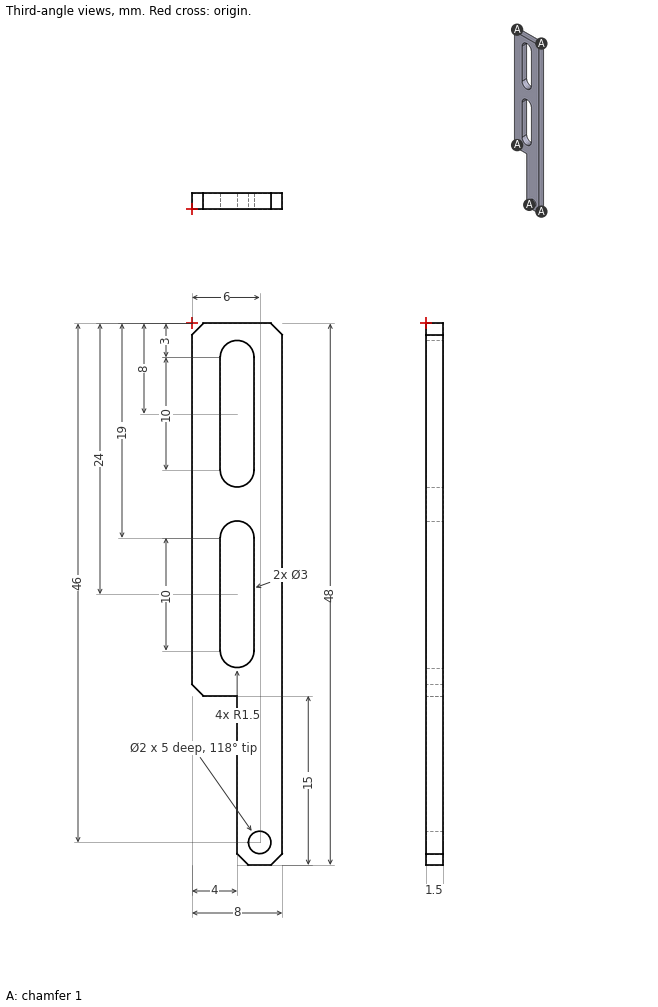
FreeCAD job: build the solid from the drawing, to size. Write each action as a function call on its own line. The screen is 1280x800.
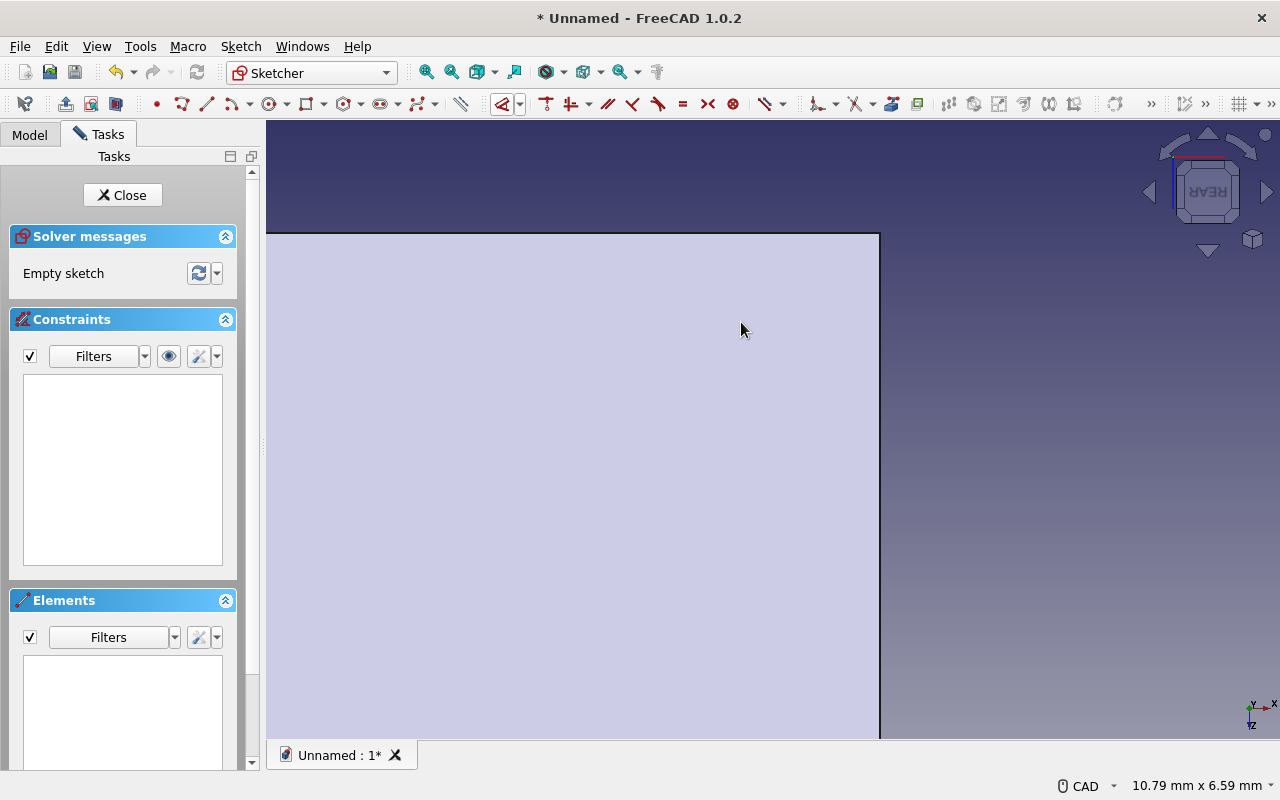
scroll(682, 414, up, 4)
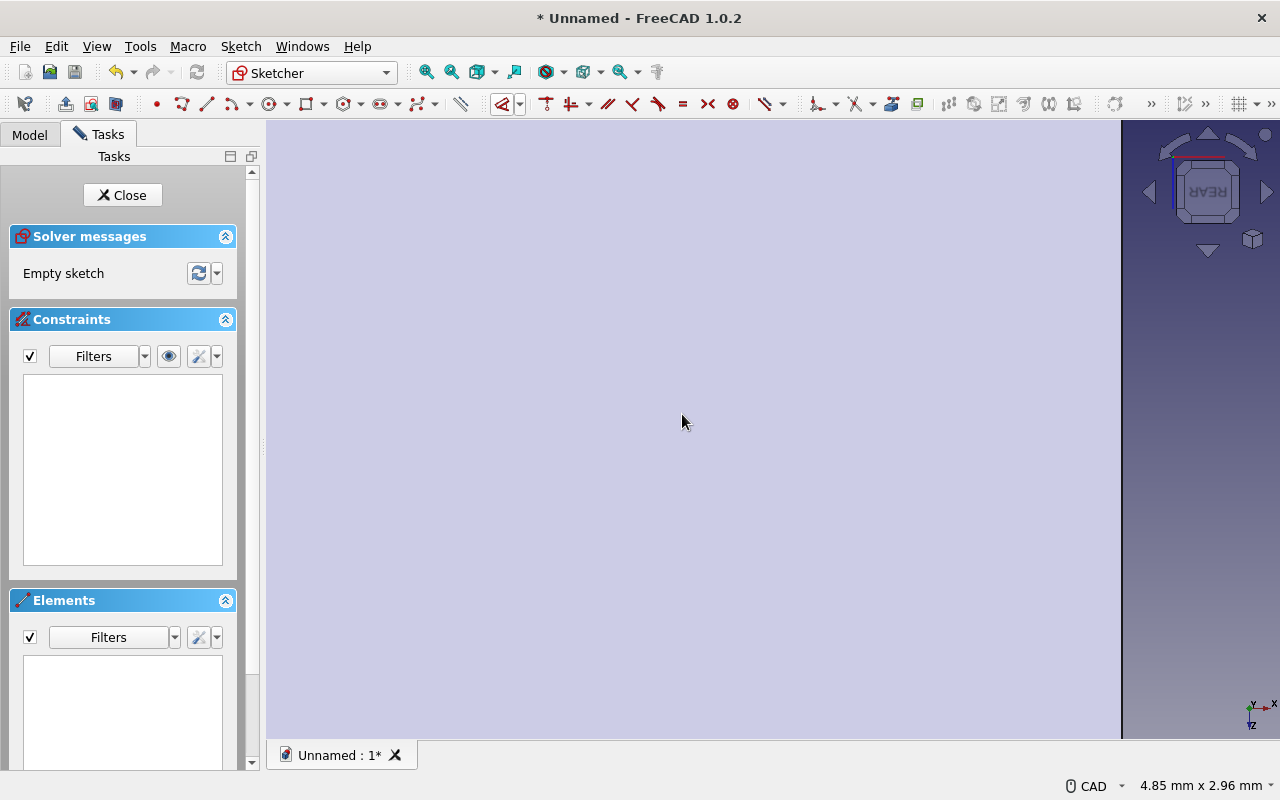
click(268, 104)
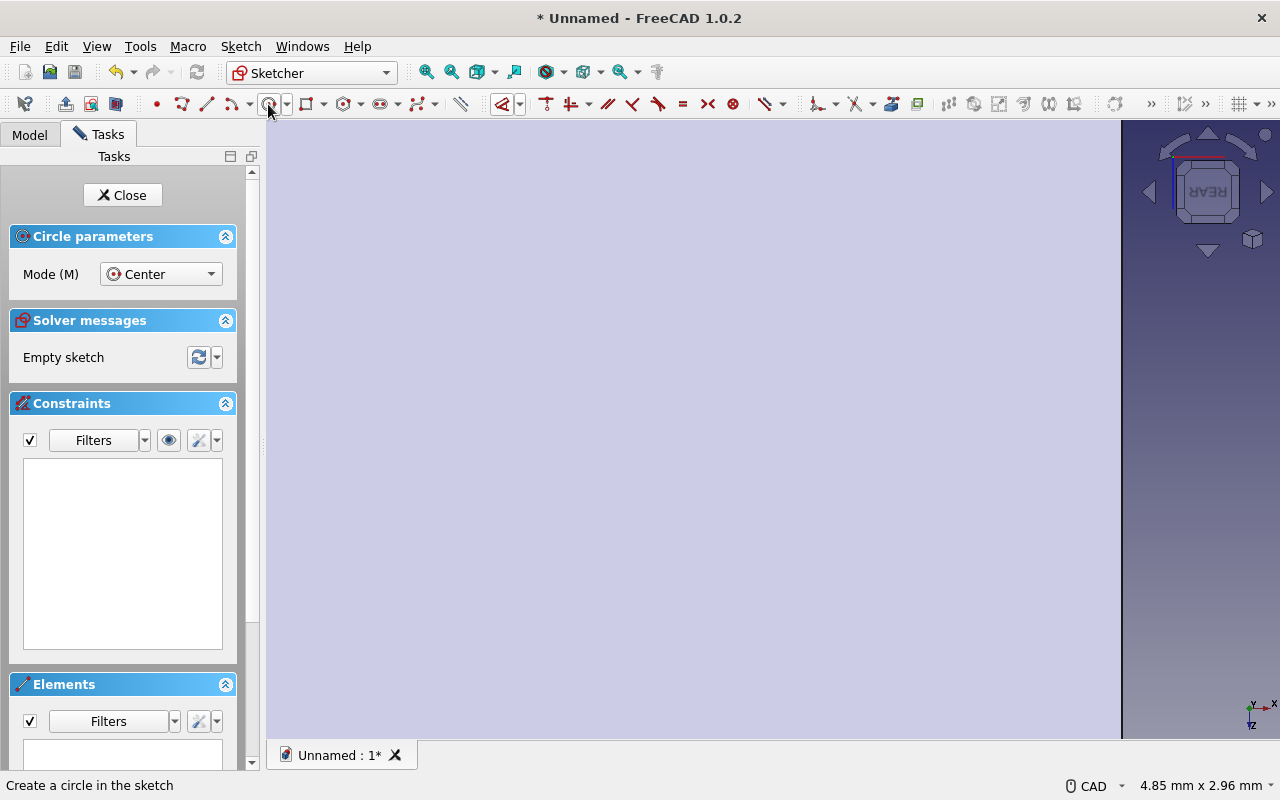
click(704, 429)
move(852, 281)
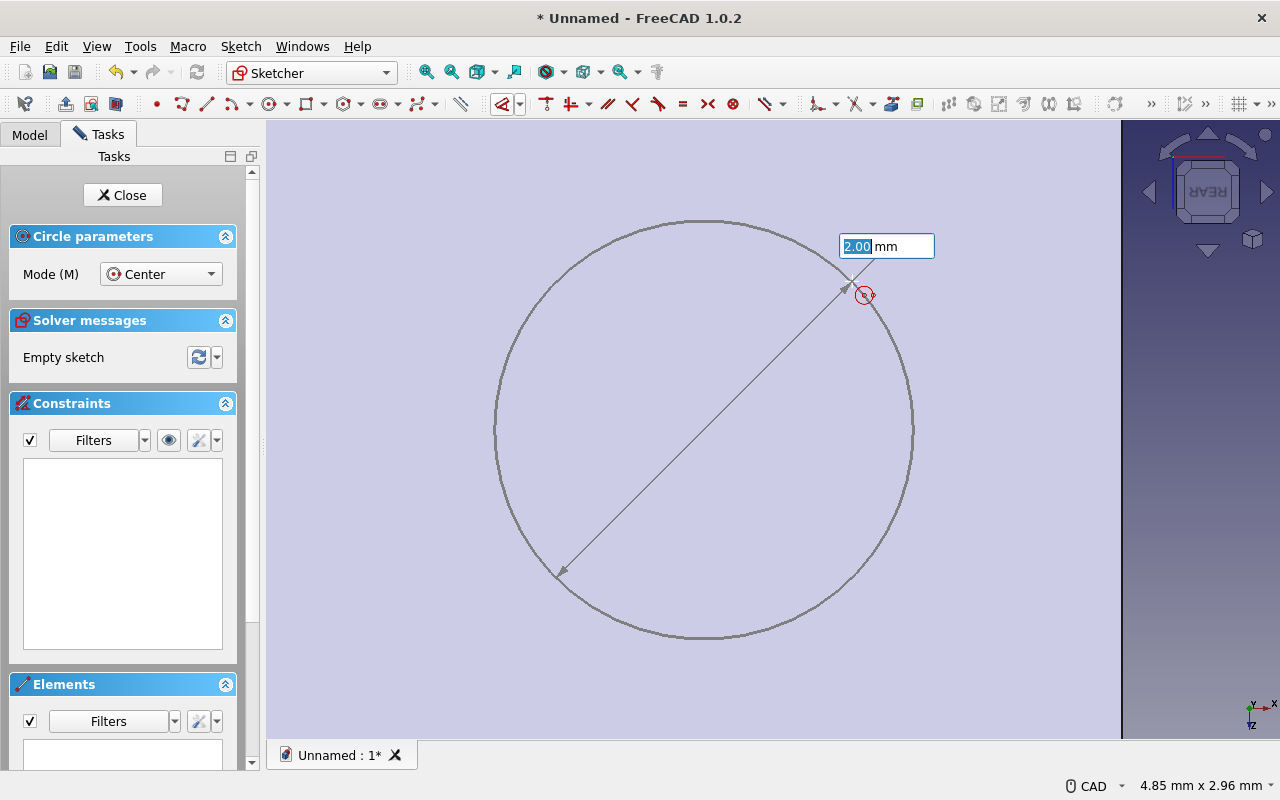
text(2)
key(Return)
key(Escape)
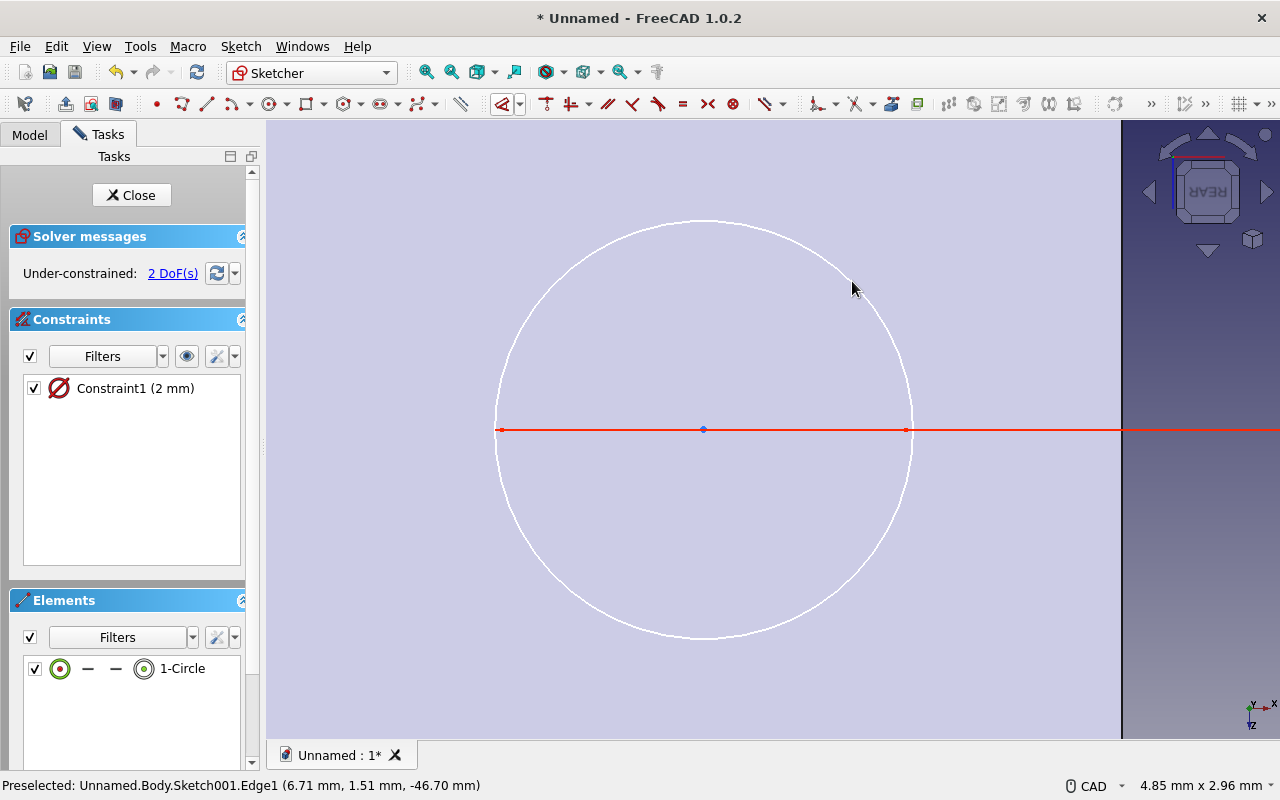
click(704, 430)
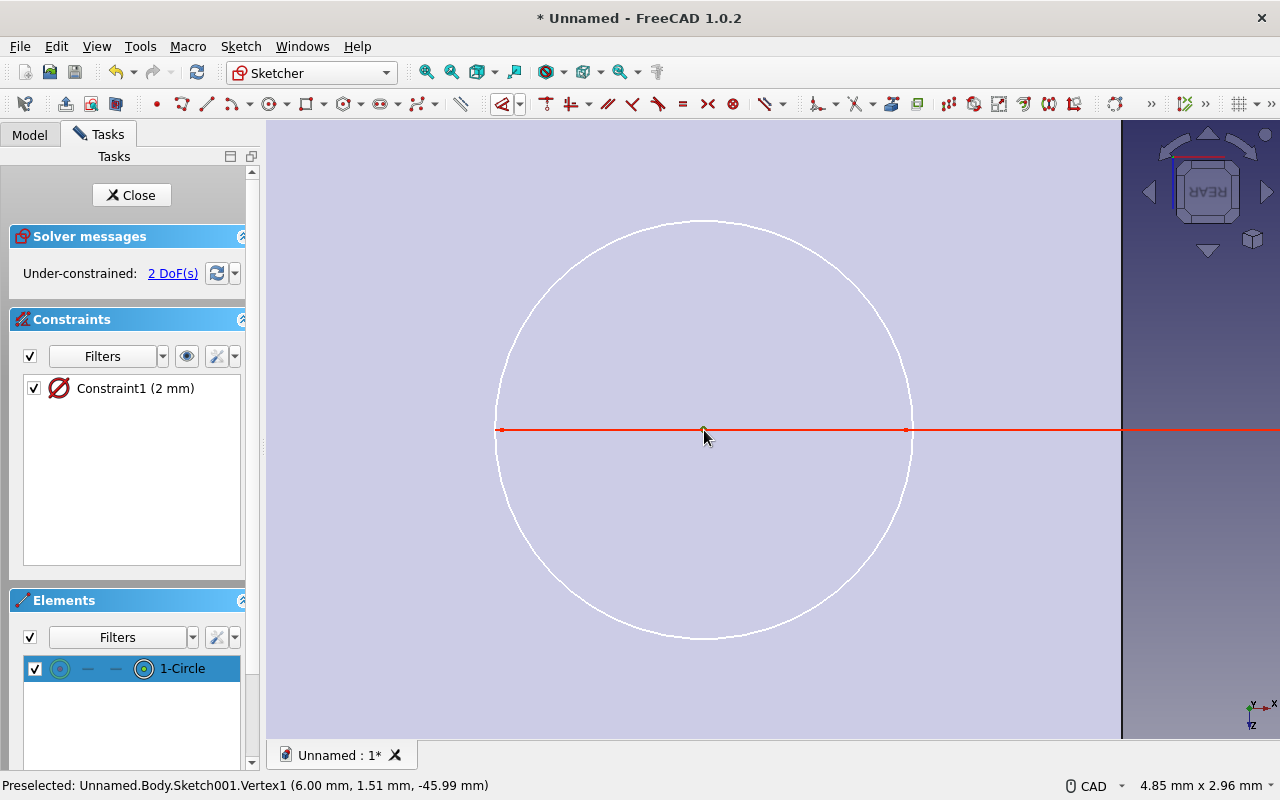
key(l)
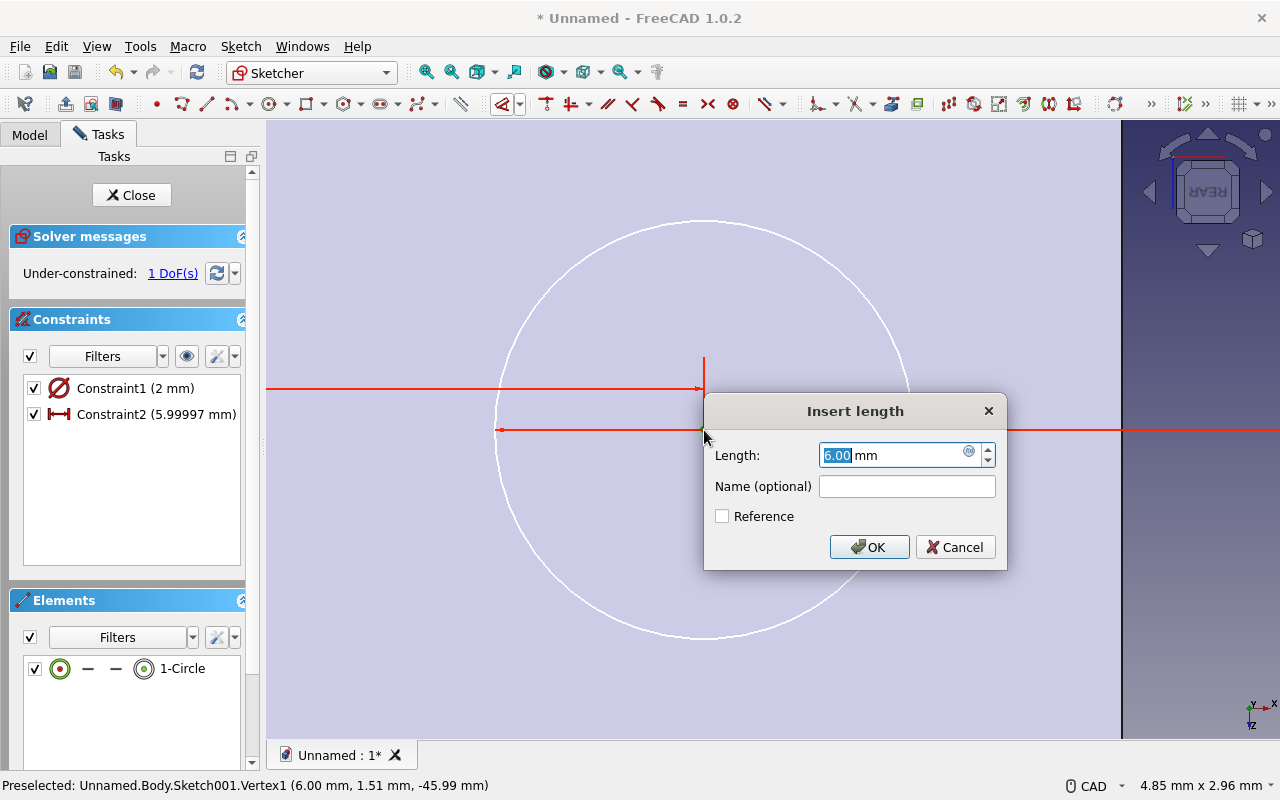
text(6)
key(Return)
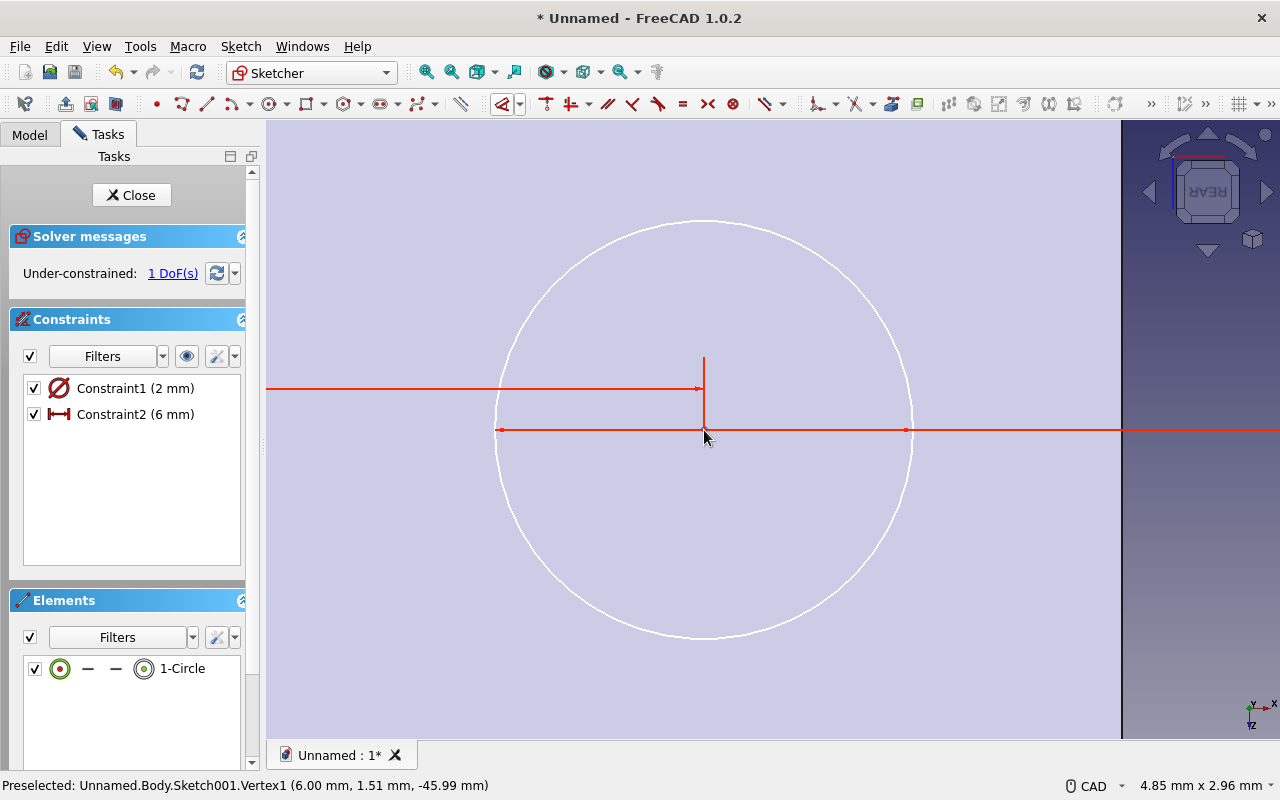
click(704, 430)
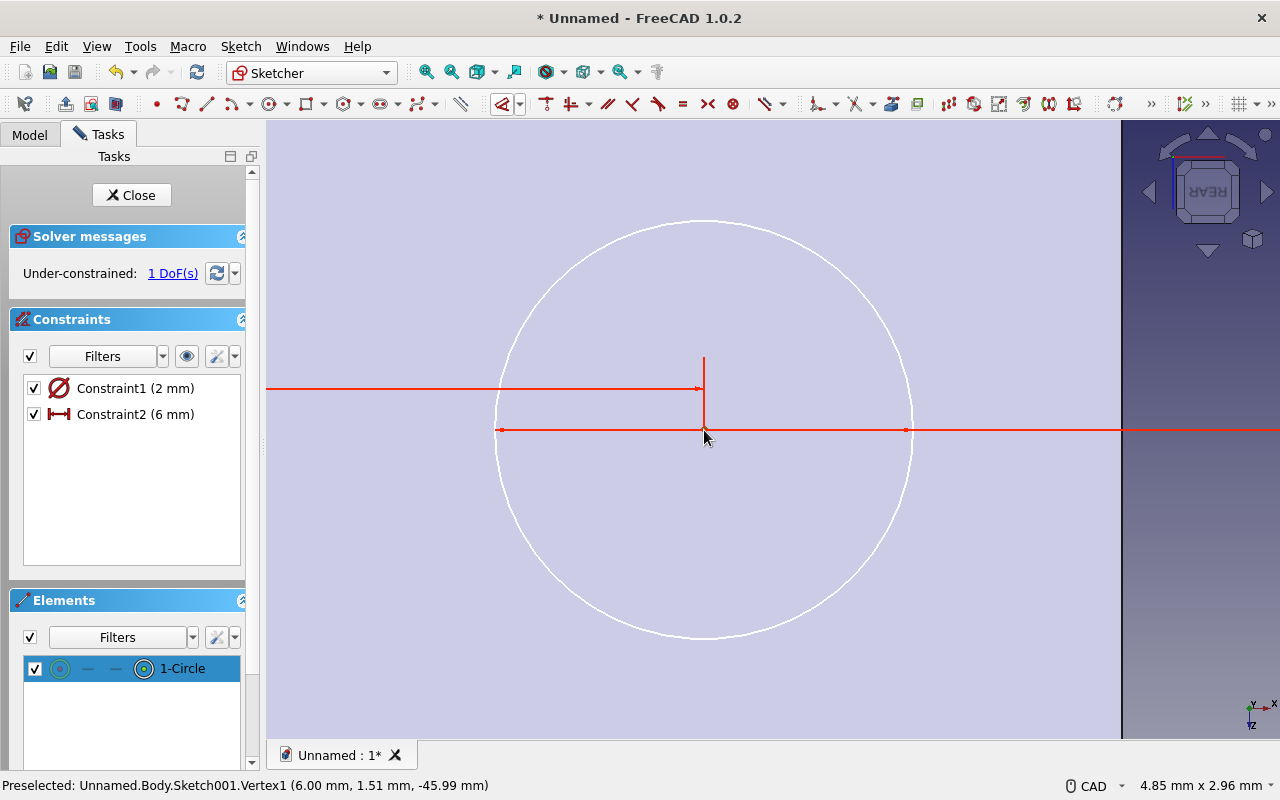
key(i)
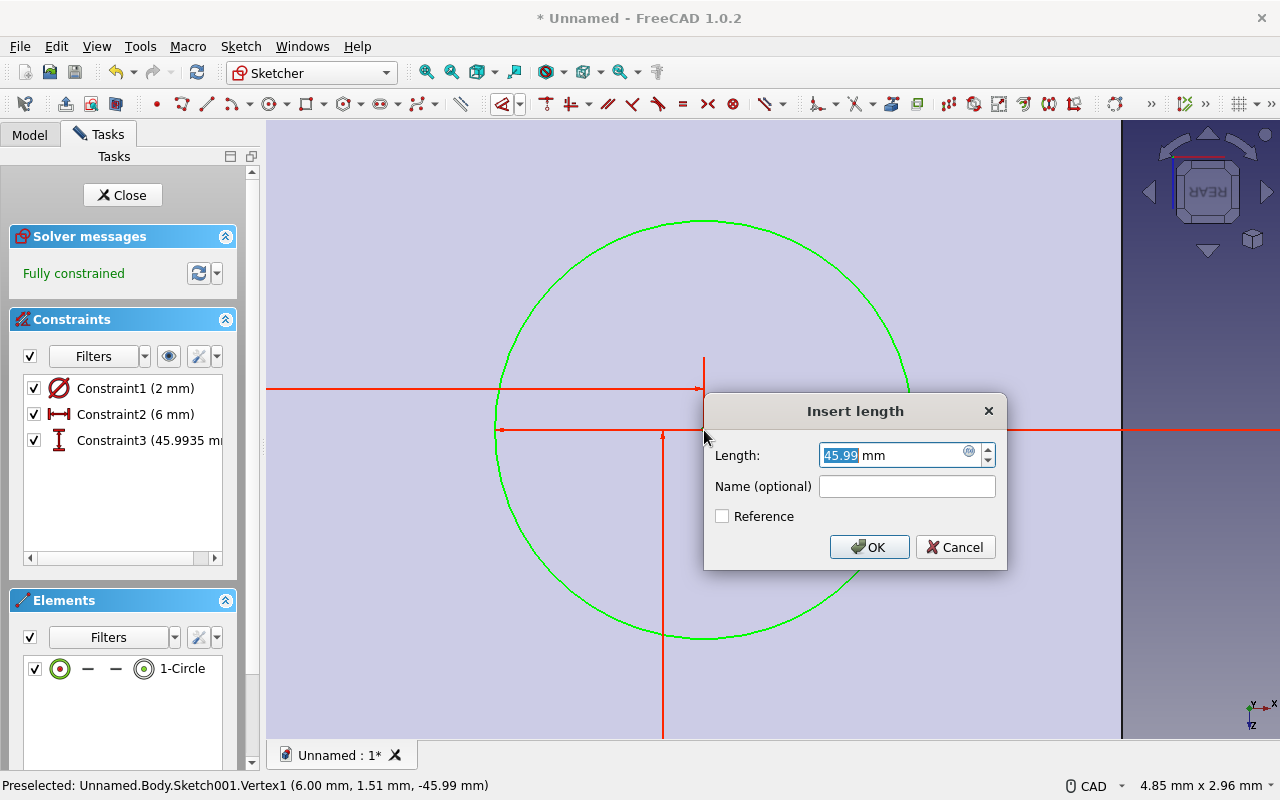
text(46)
key(Return)